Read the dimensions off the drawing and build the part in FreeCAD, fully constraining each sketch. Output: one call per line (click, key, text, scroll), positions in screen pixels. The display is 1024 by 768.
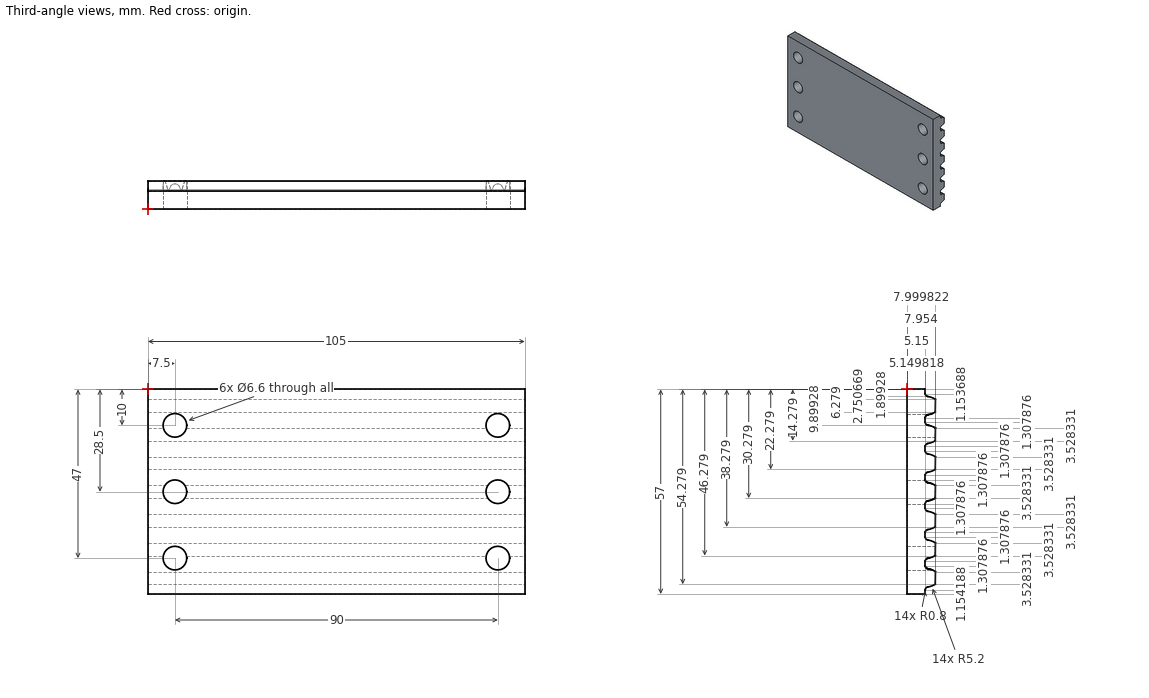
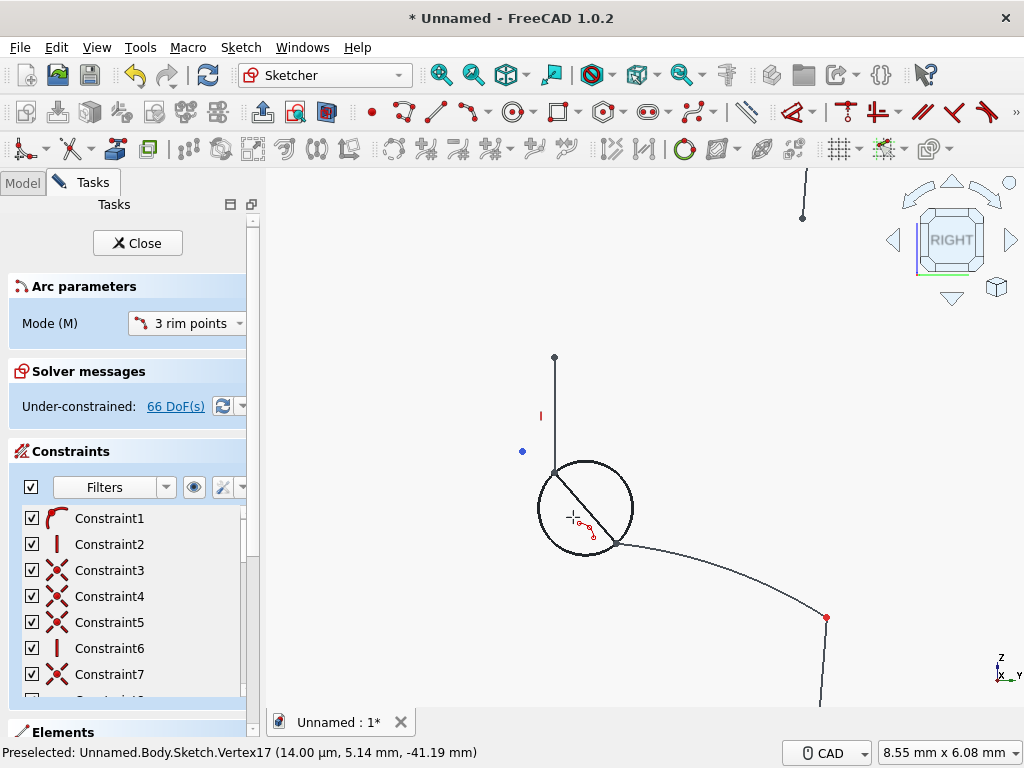
click(573, 516)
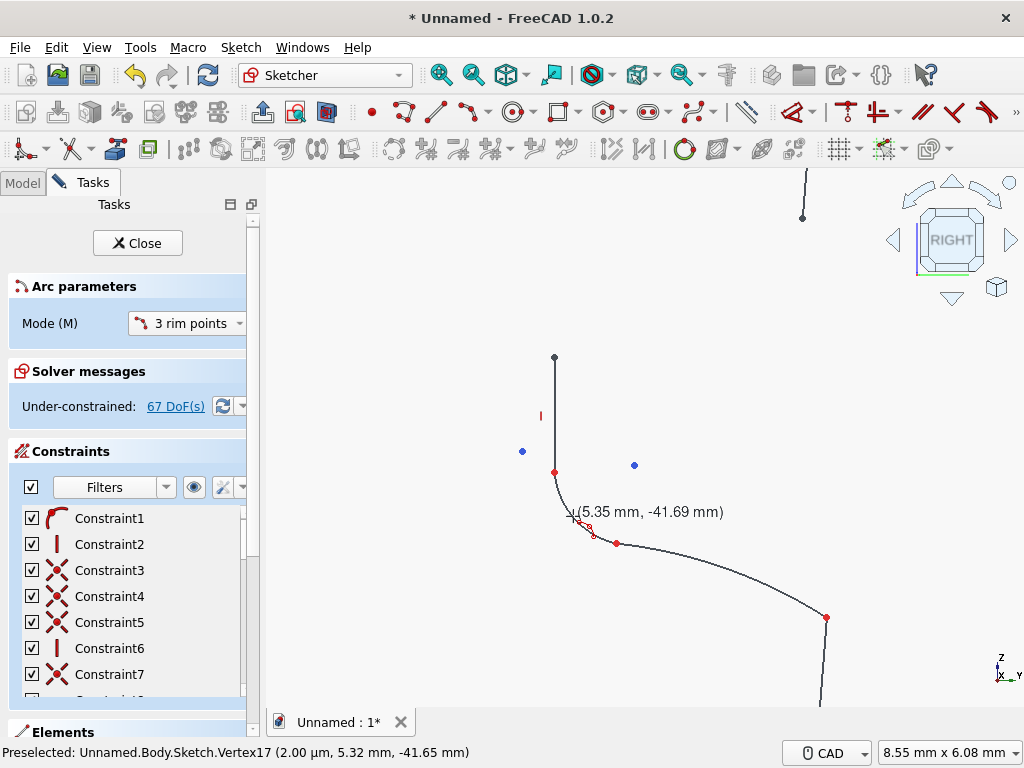
scroll(586, 525, down, 13)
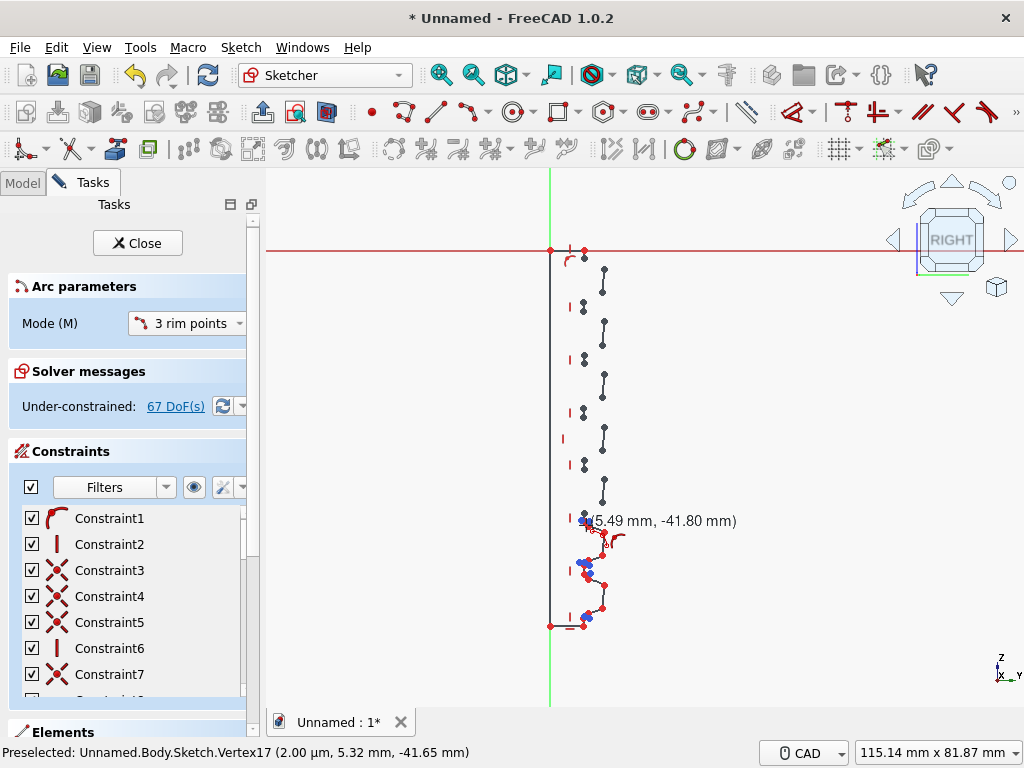
scroll(584, 513, up, 7)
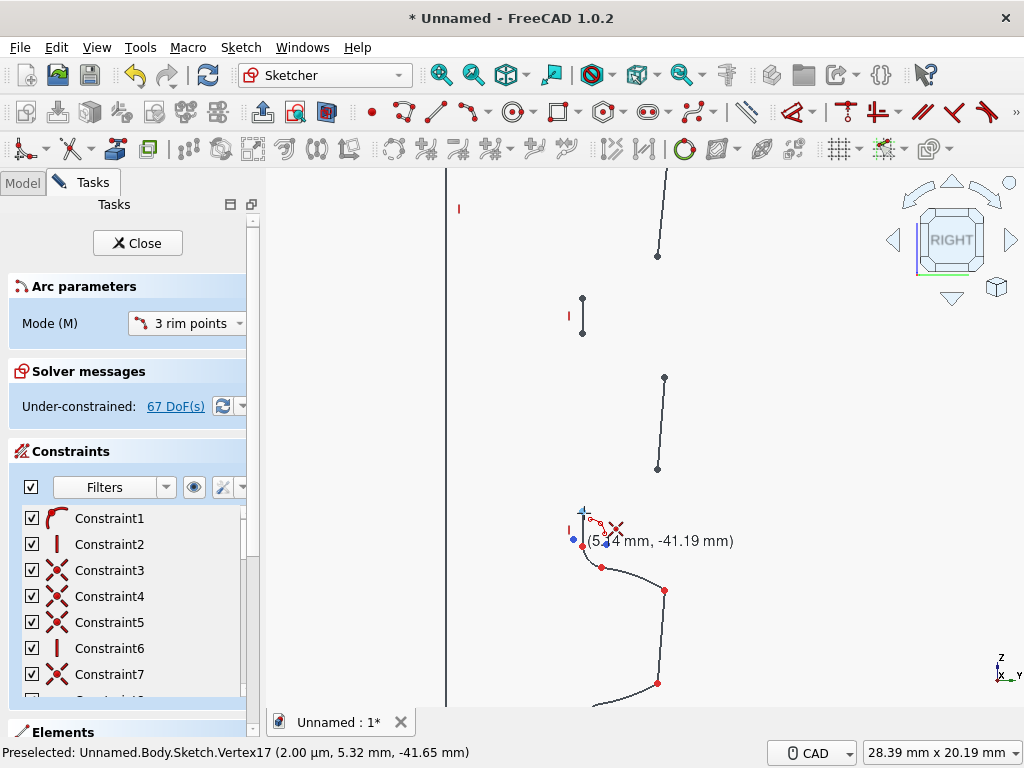
click(583, 512)
click(602, 489)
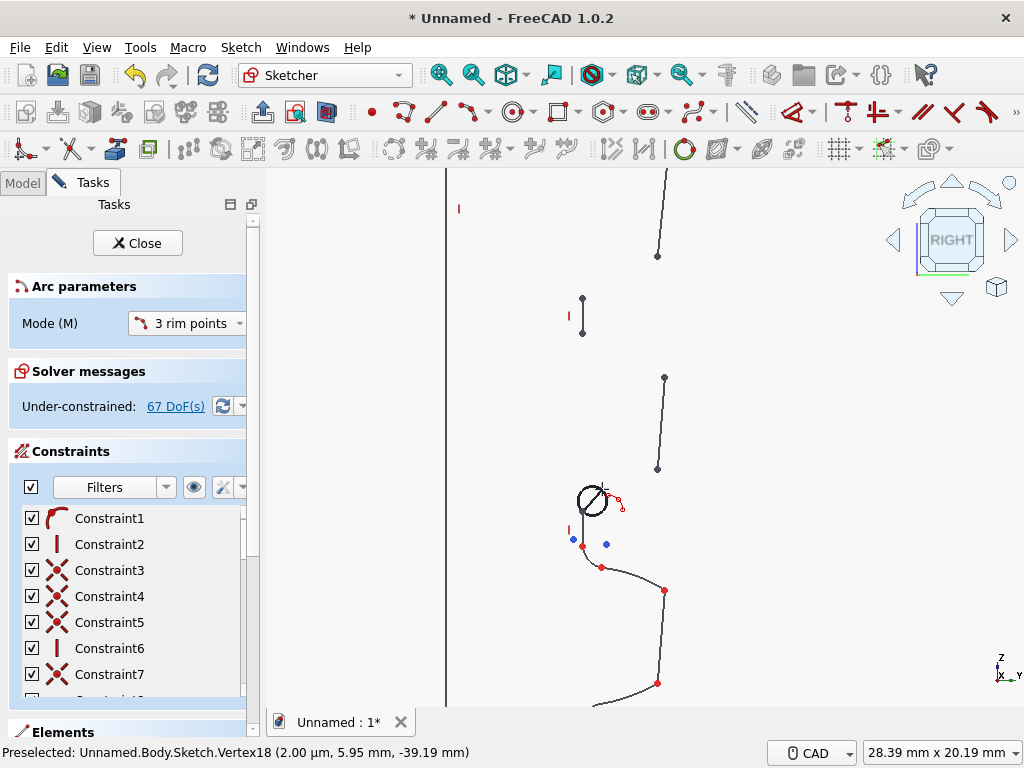
scroll(589, 496, up, 6)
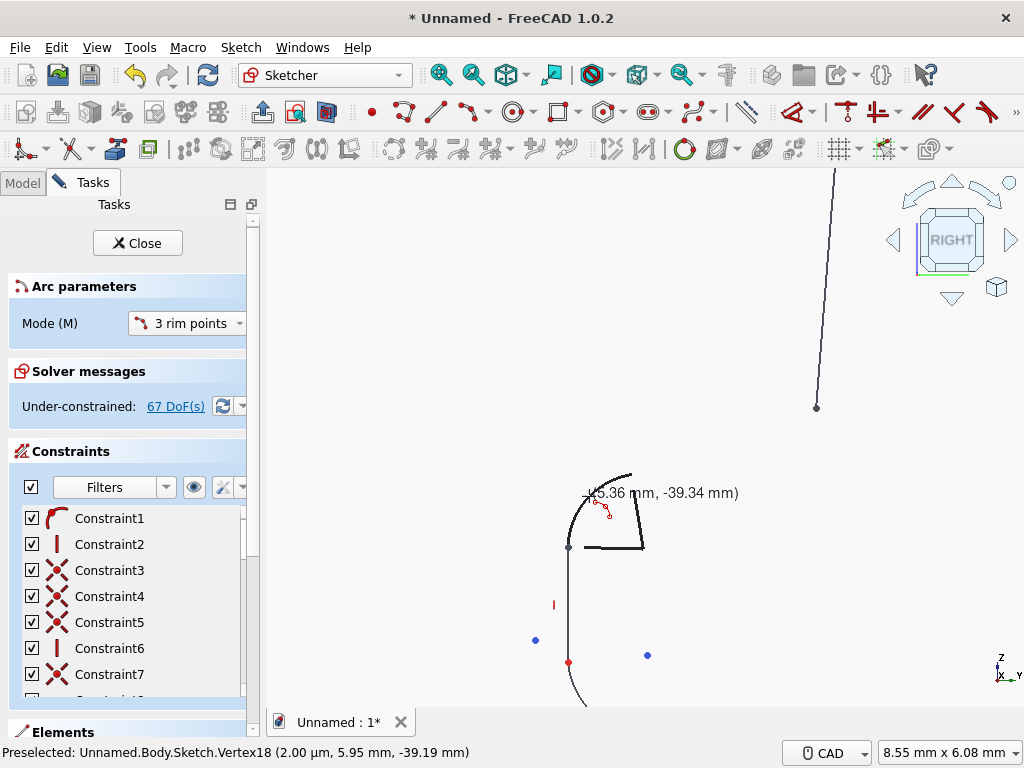
click(587, 496)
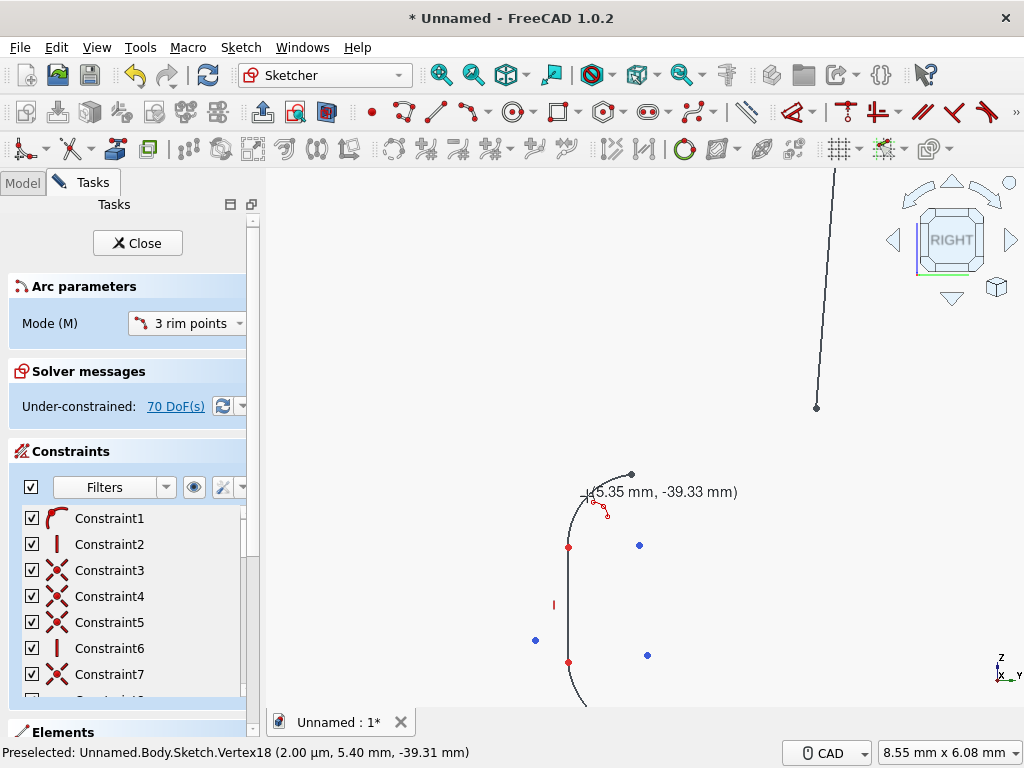
scroll(585, 510, down, 13)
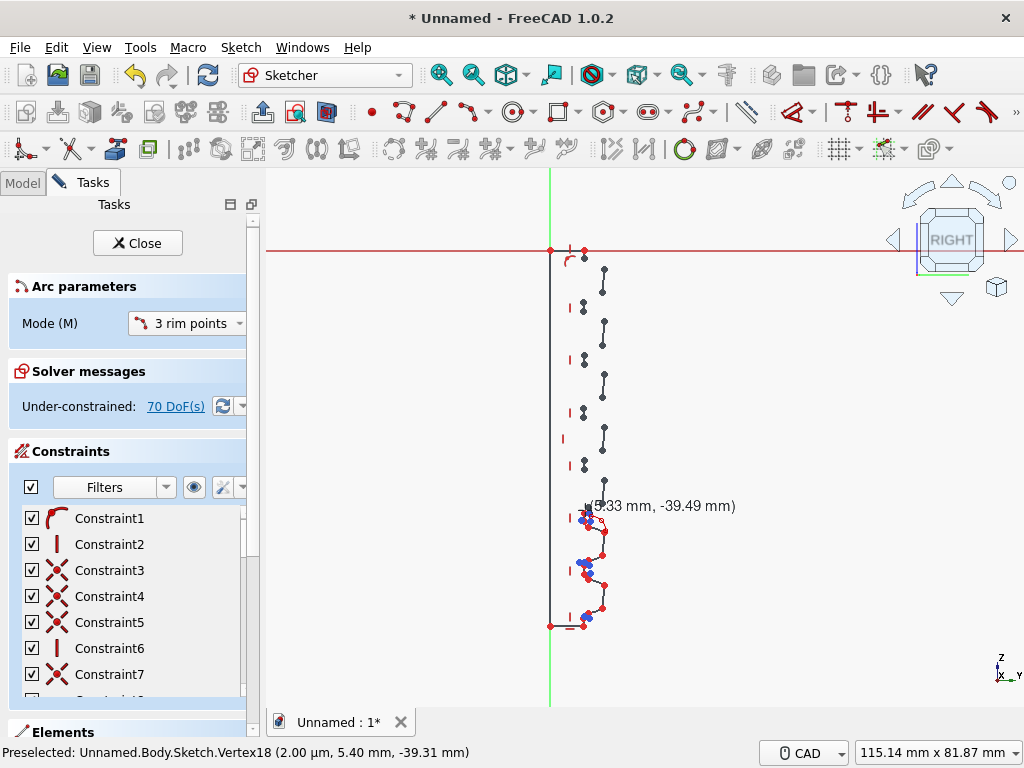
scroll(589, 508, up, 6)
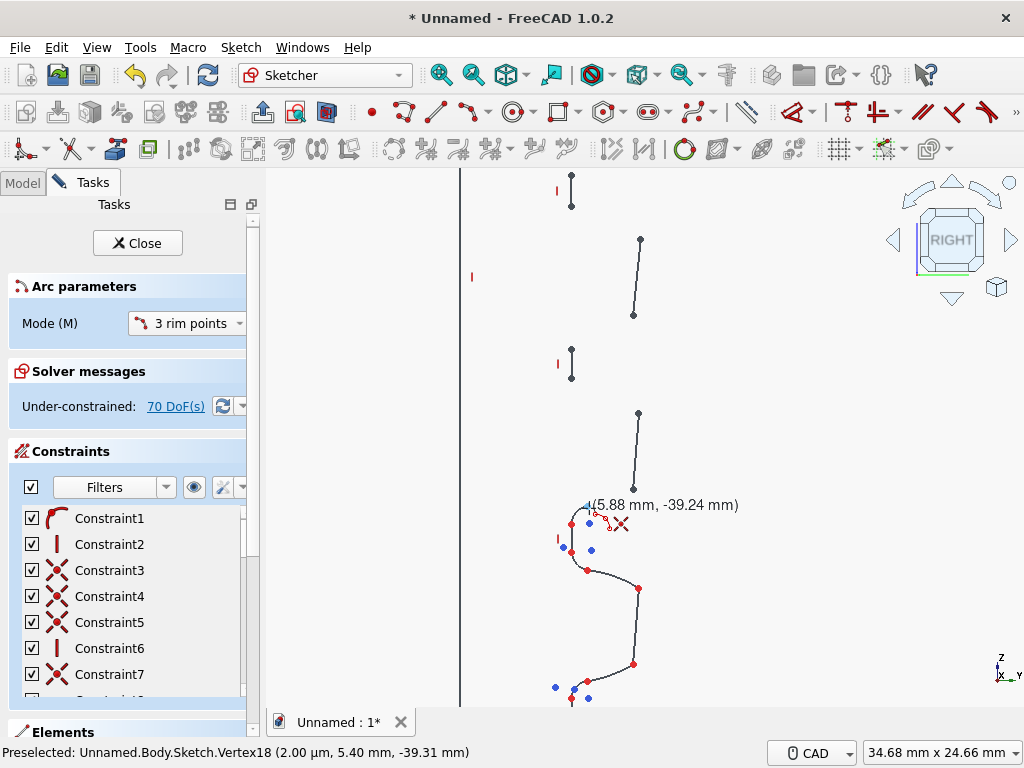
click(587, 506)
click(633, 490)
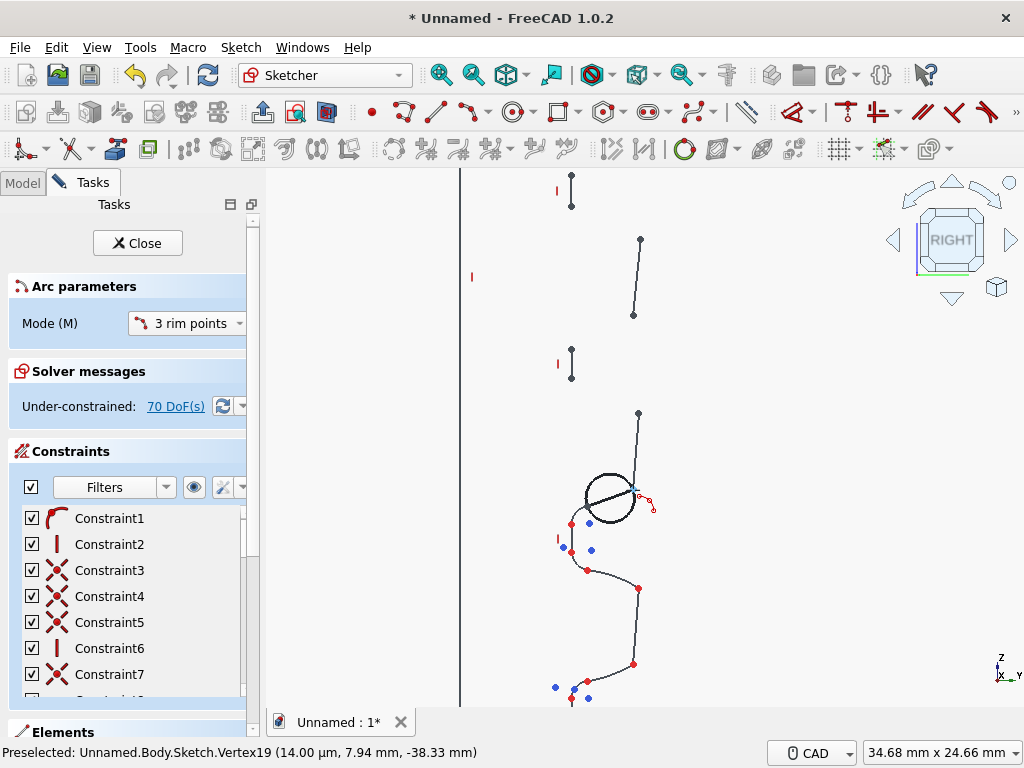
scroll(611, 500, up, 9)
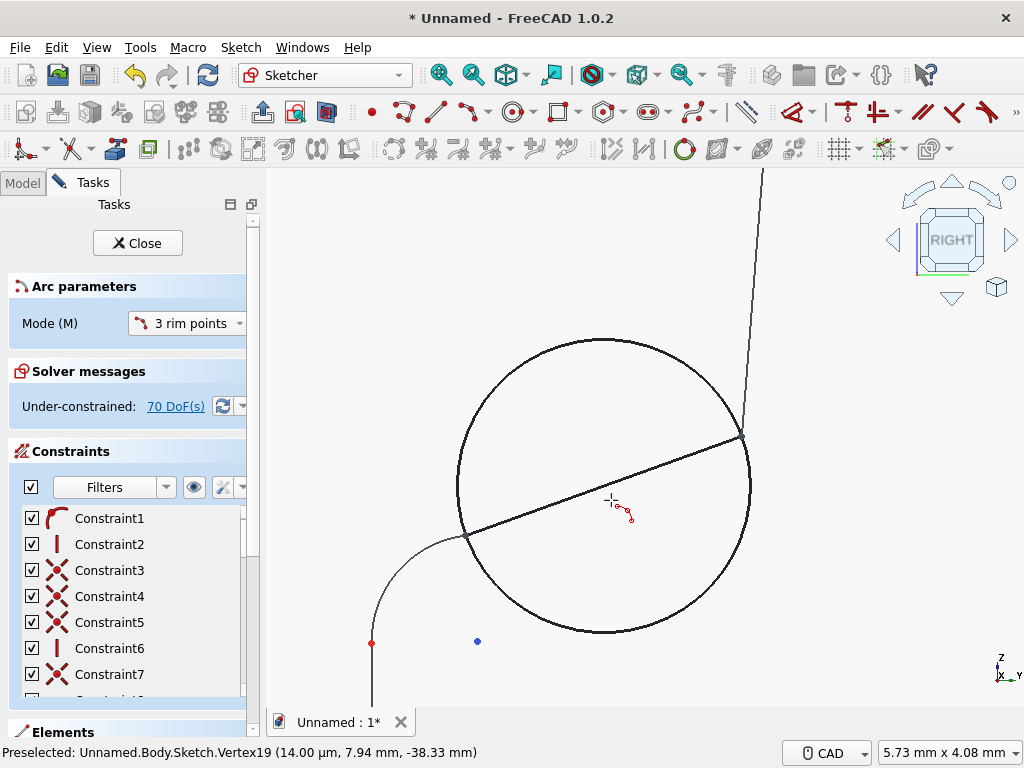
click(610, 496)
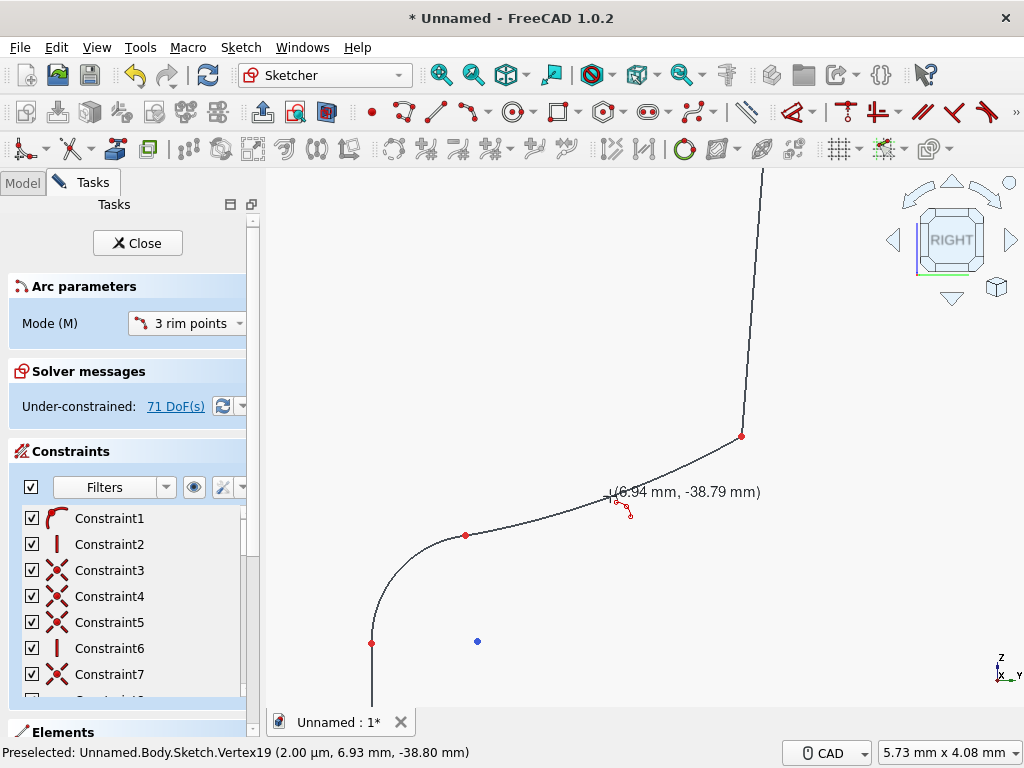
scroll(595, 506, down, 15)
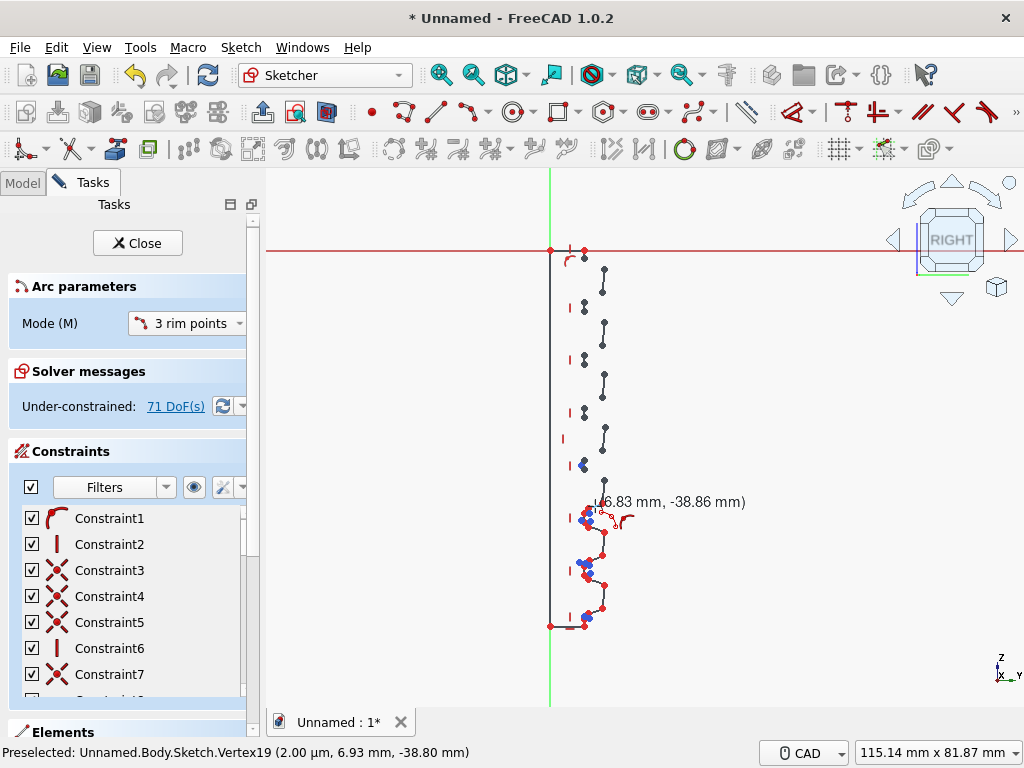
scroll(603, 480, up, 2)